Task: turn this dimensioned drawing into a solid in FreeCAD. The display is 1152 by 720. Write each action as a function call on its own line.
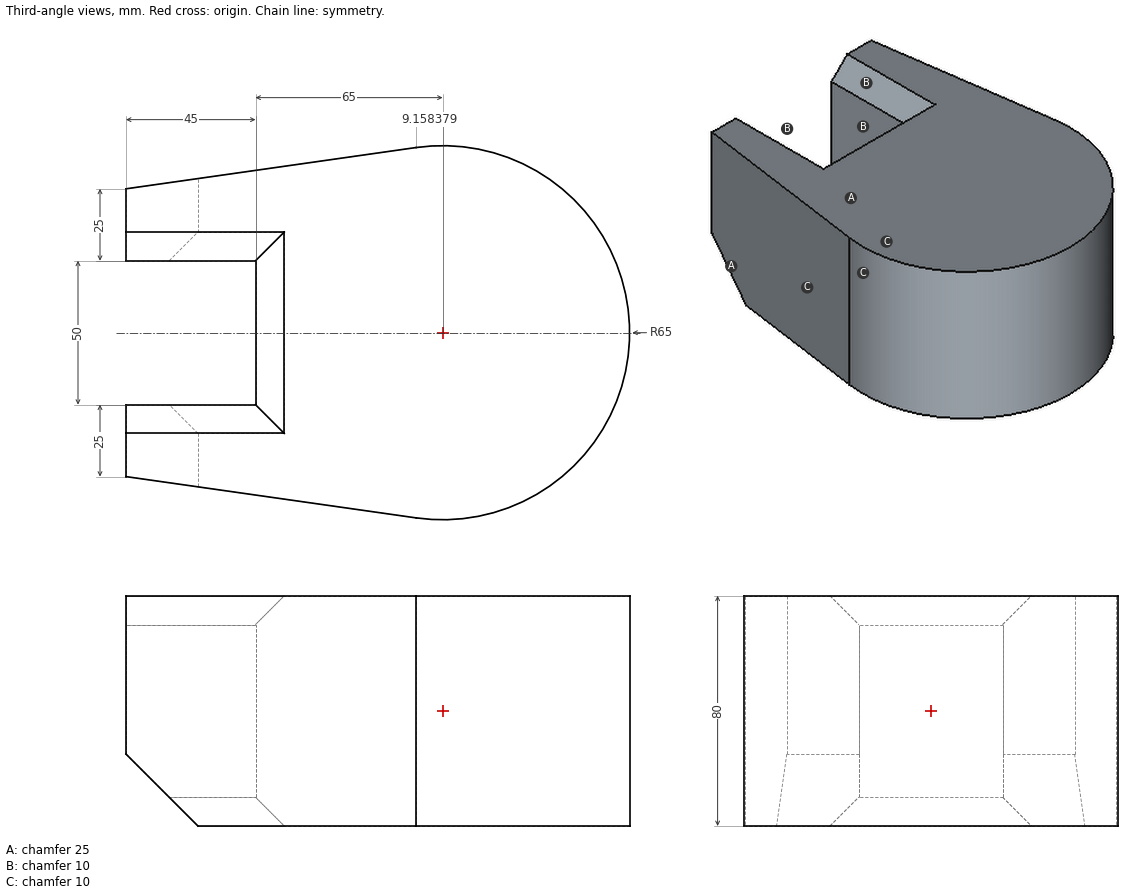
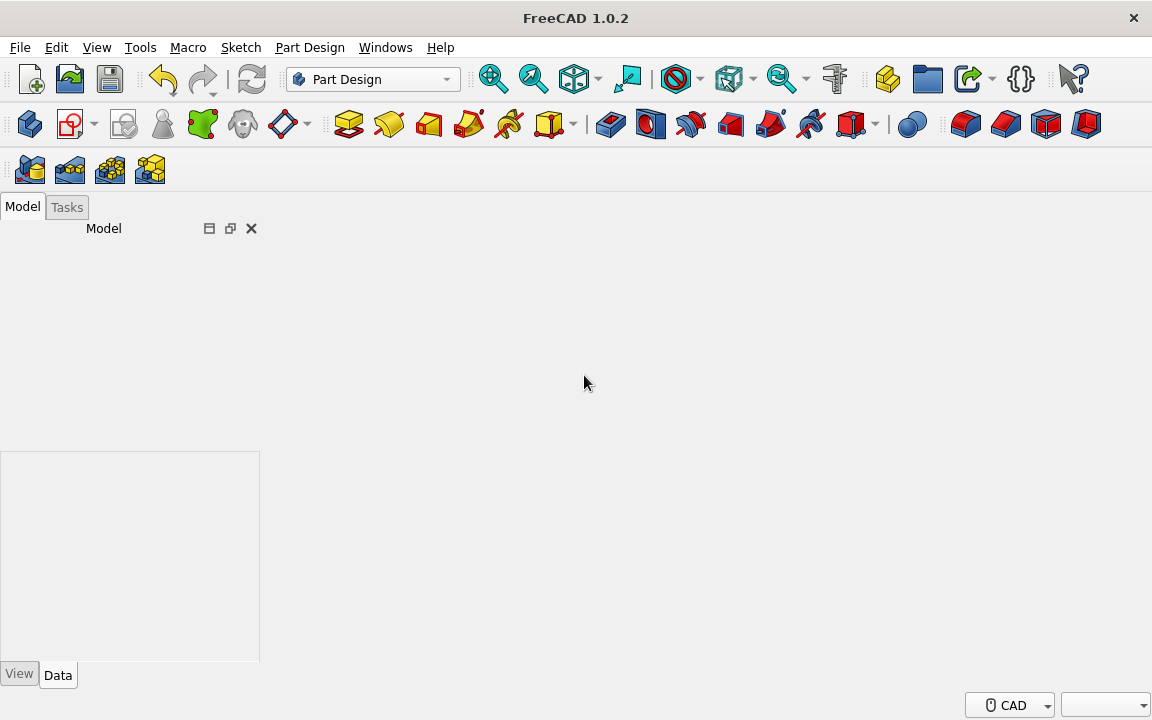
click(30, 80)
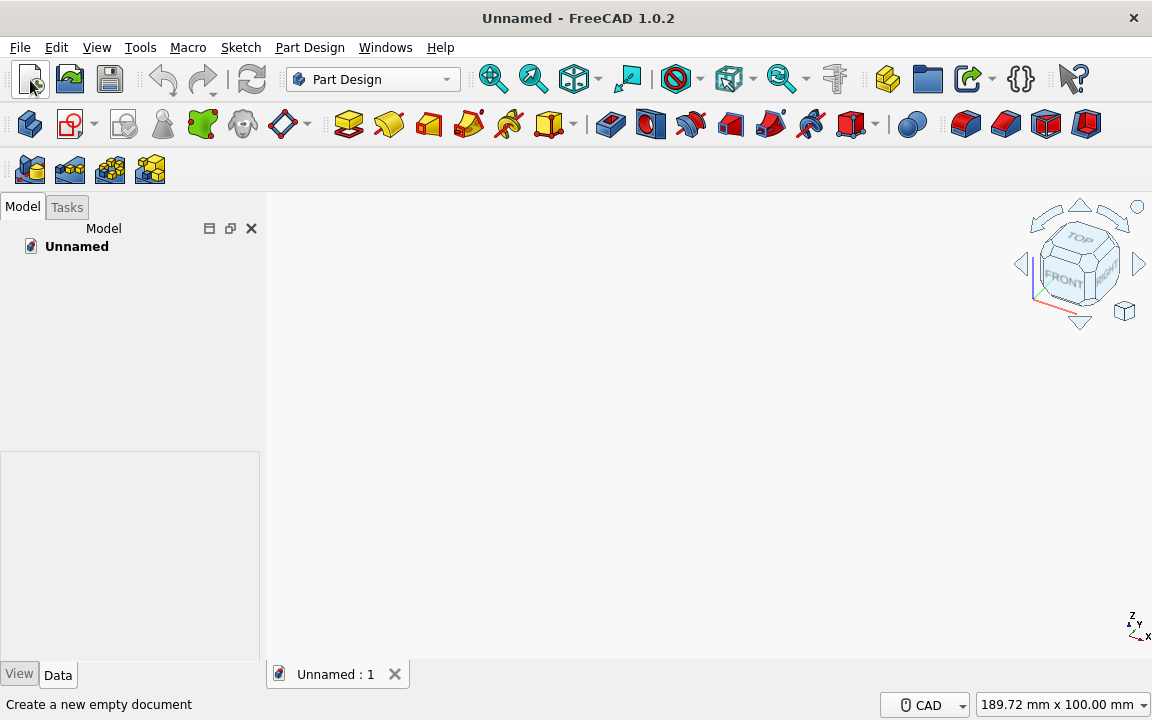
click(70, 124)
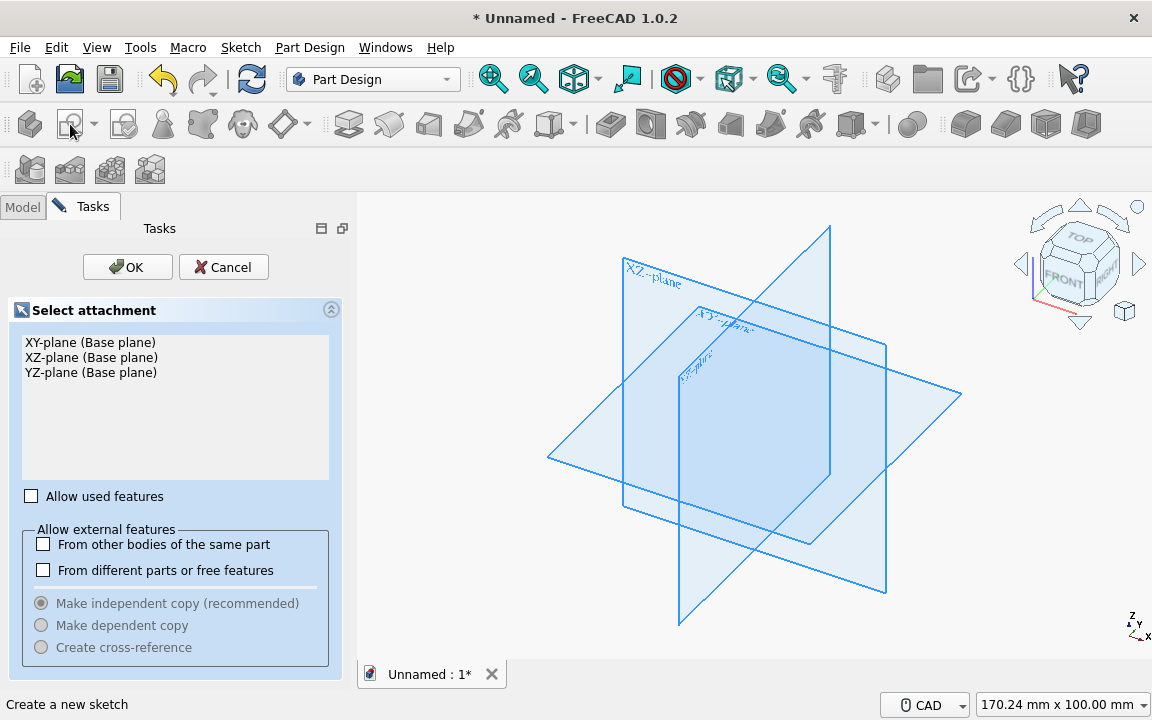
click(82, 342)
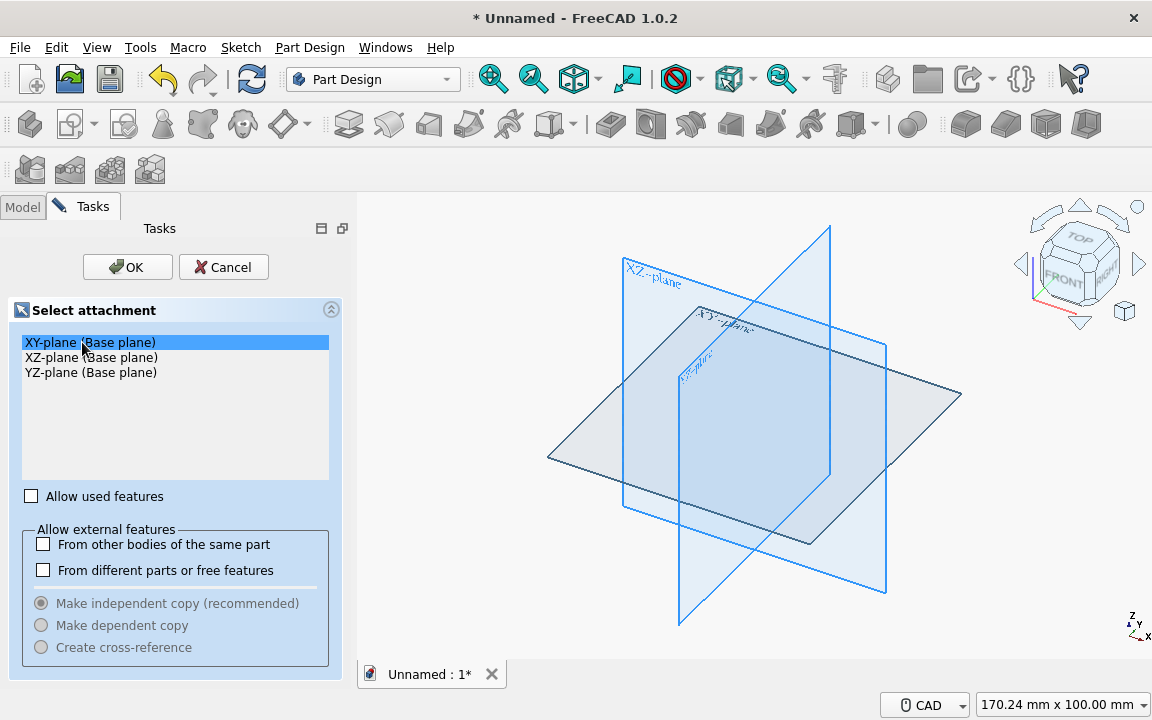
click(128, 267)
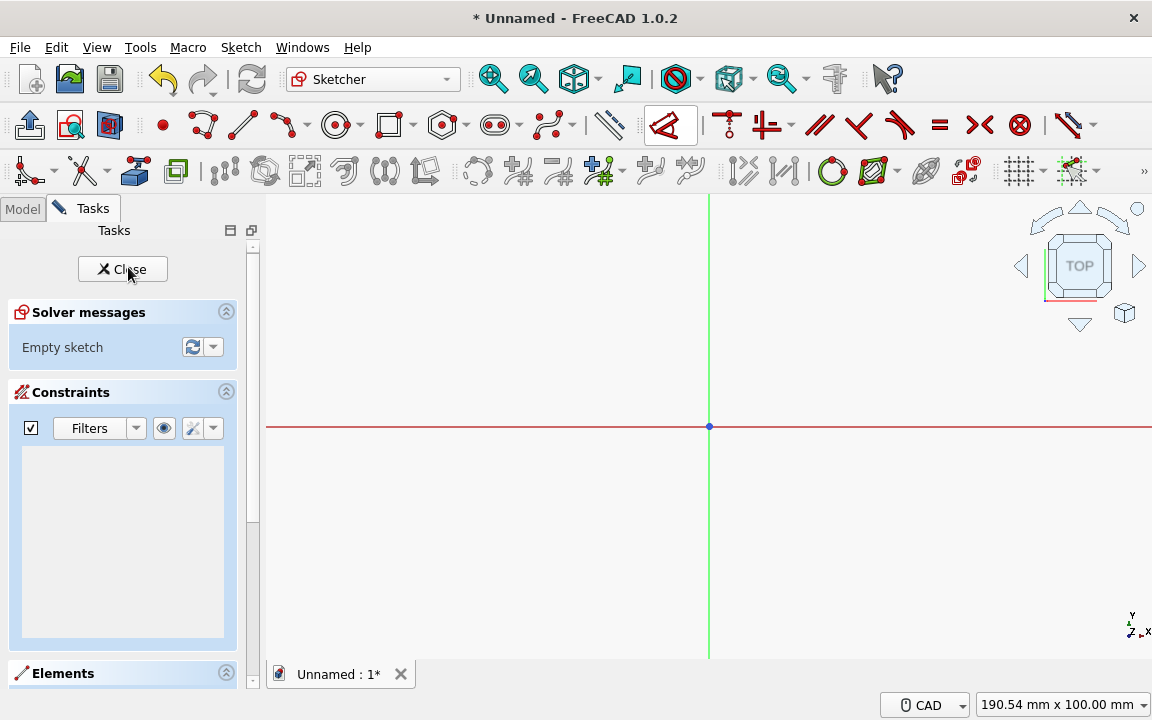
scroll(670, 426, down, 4)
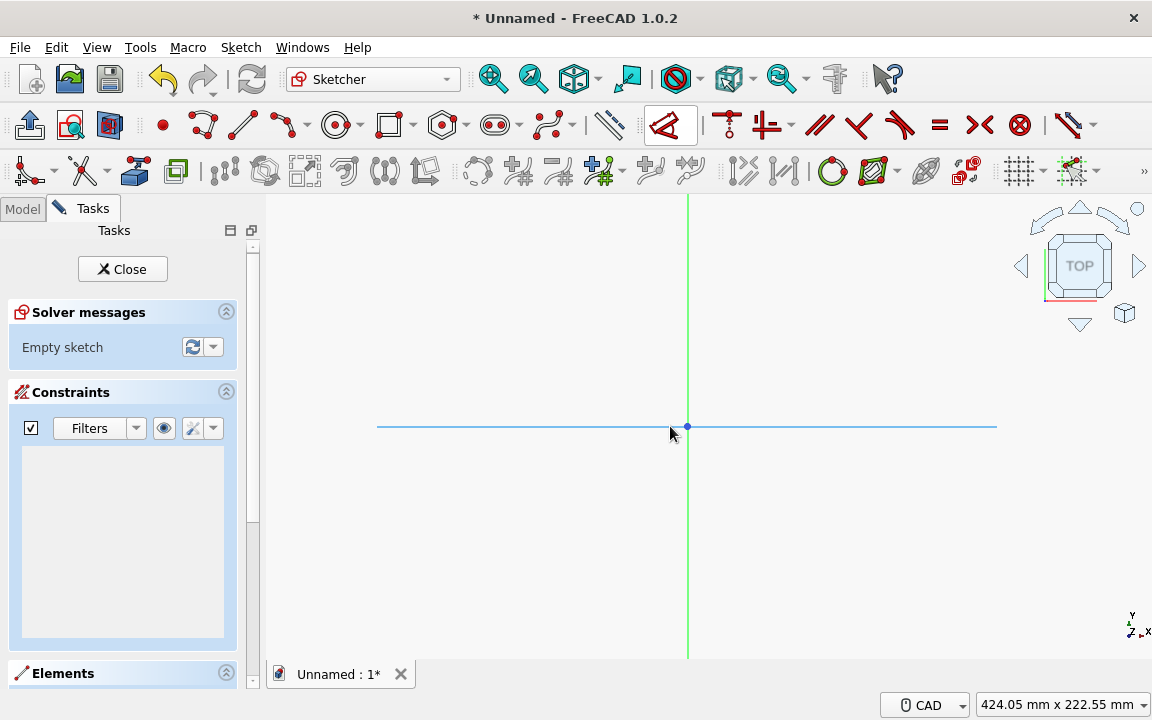
click(204, 126)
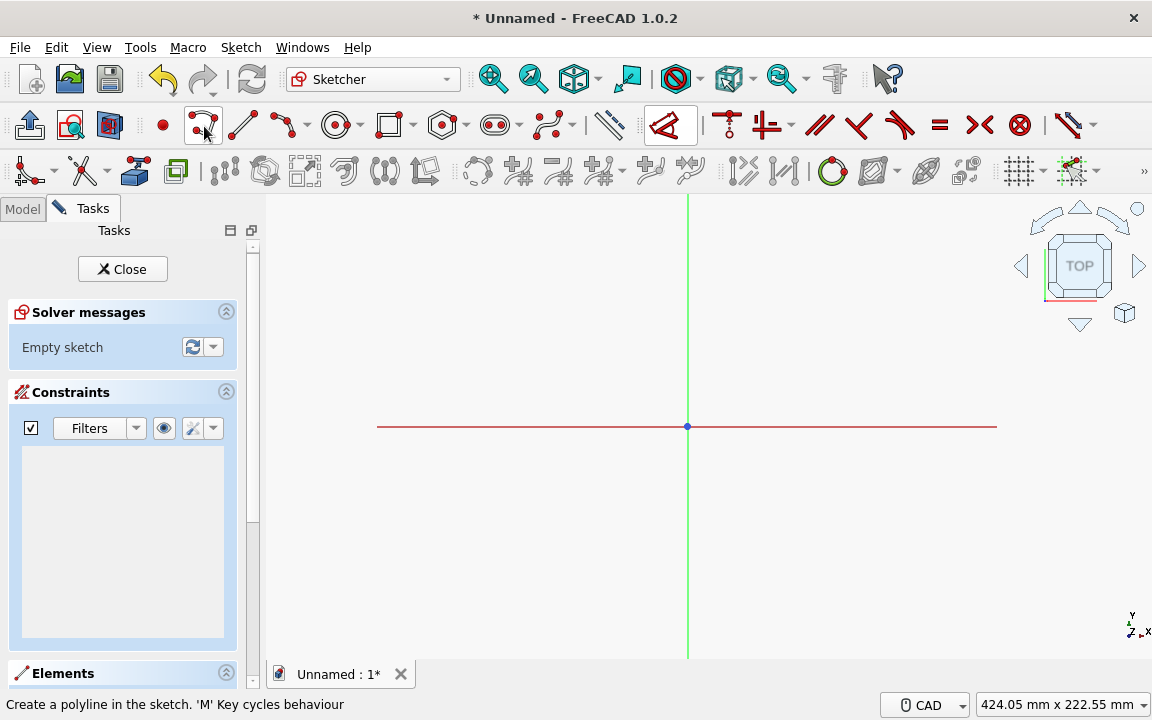
click(669, 292)
click(458, 322)
click(458, 374)
click(552, 374)
click(552, 479)
click(458, 479)
click(458, 531)
click(669, 561)
right_click(669, 561)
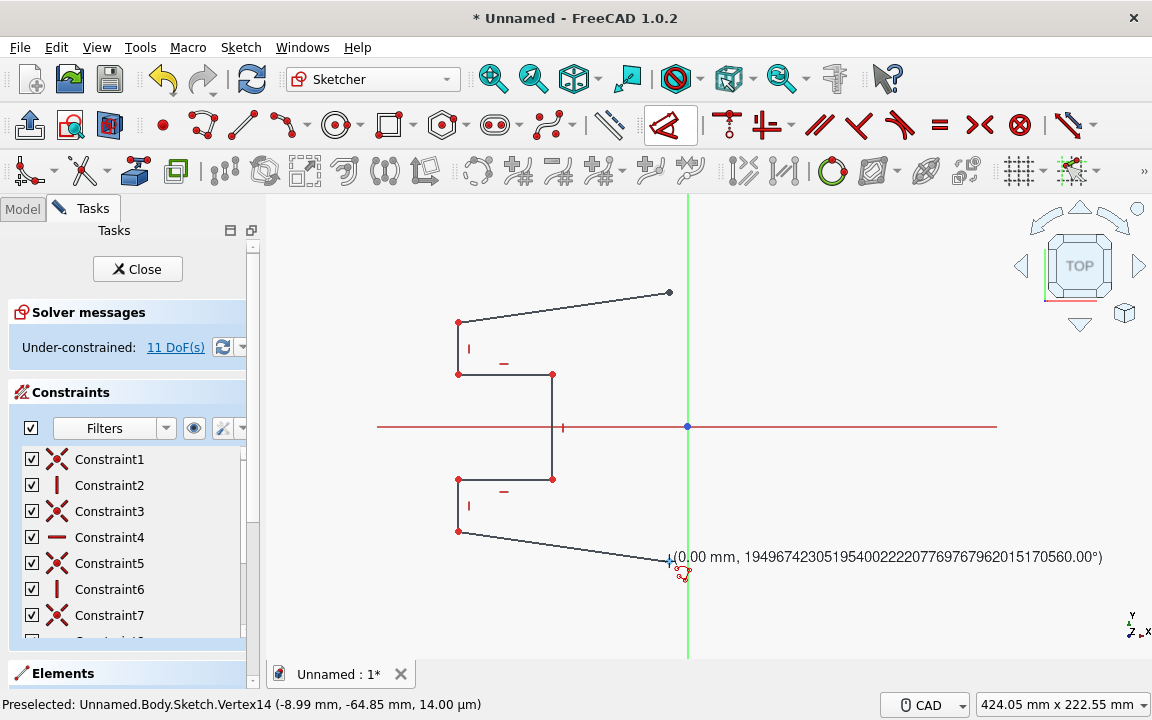
click(284, 126)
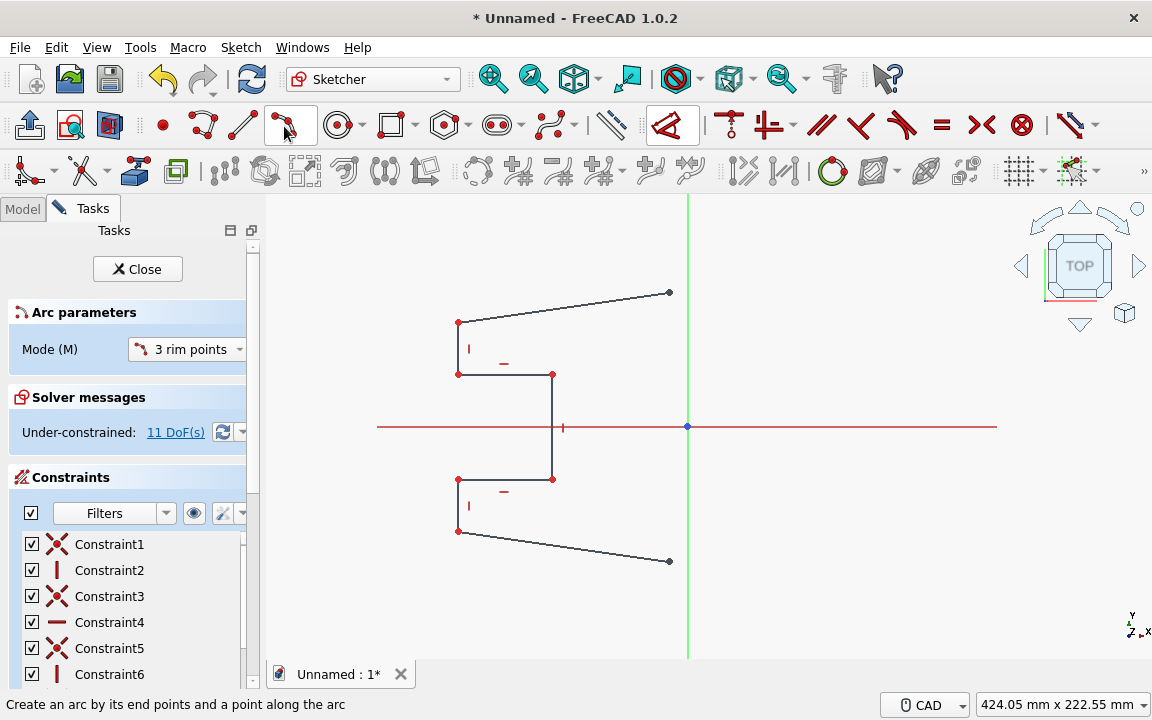
click(669, 562)
click(669, 293)
click(816, 472)
key(Escape)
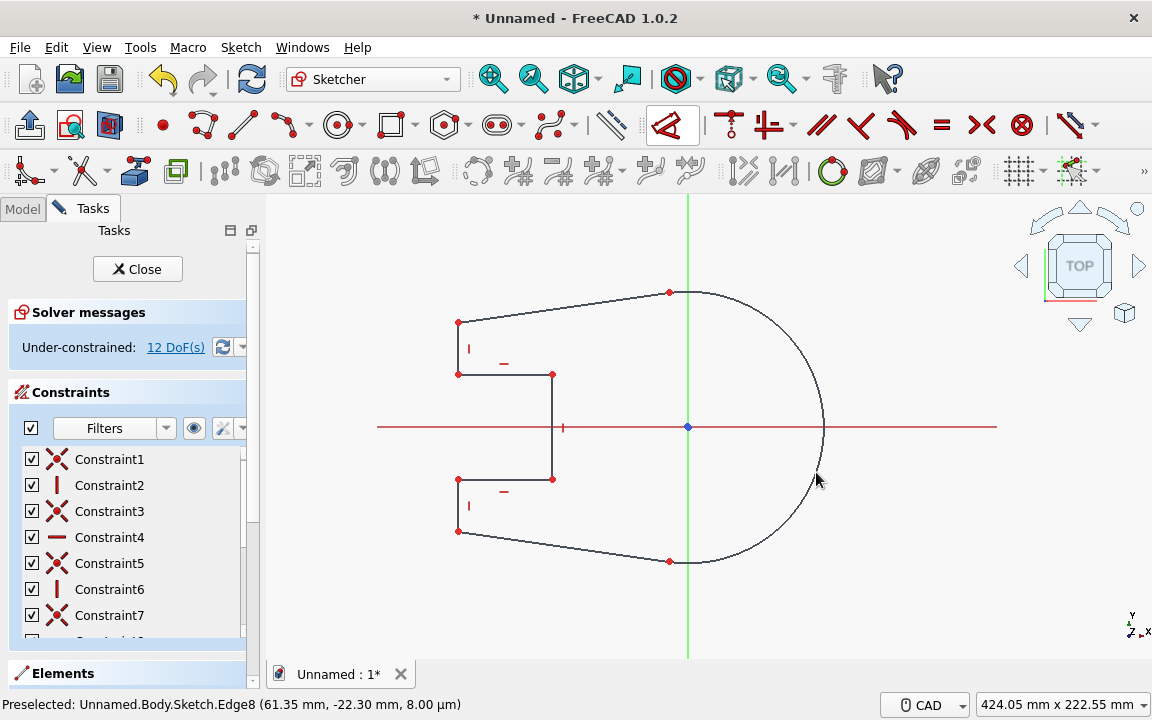
drag(678, 416, 698, 438)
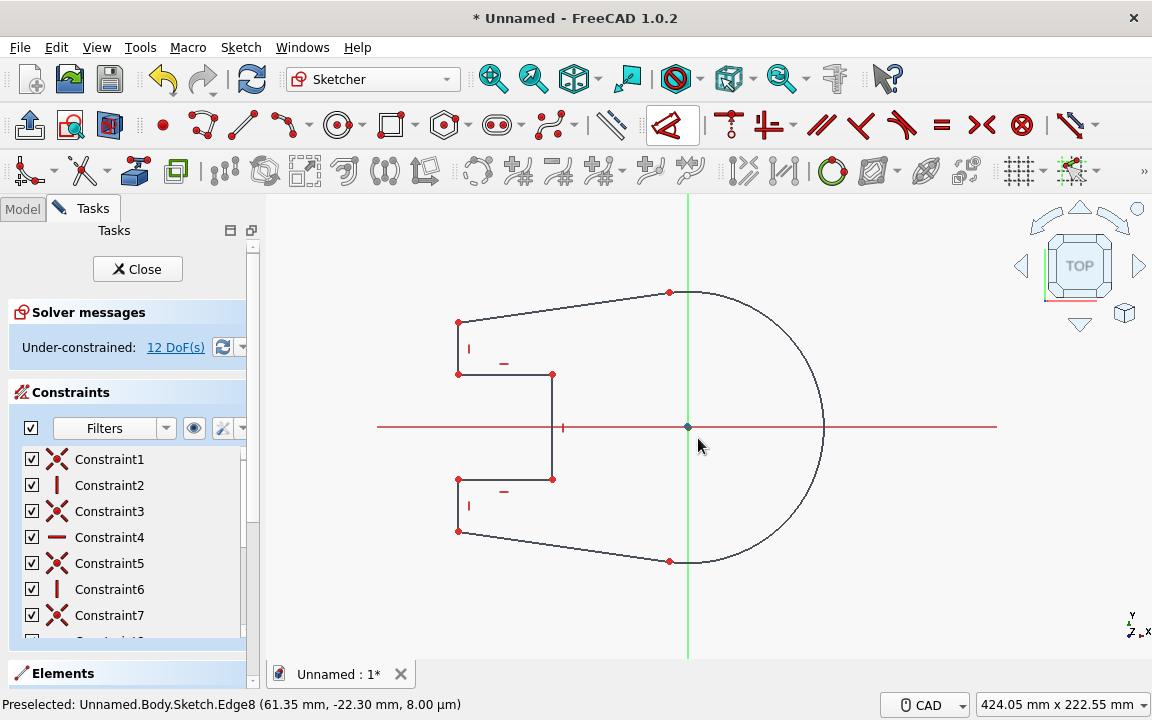
key(c)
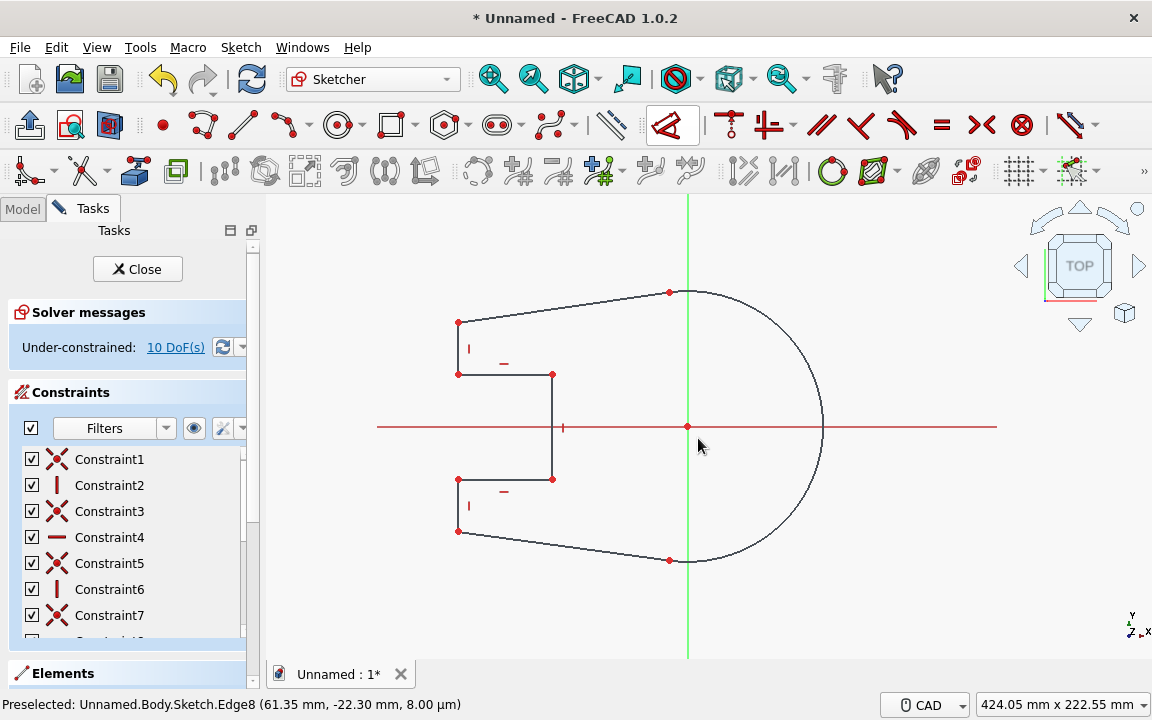
click(458, 375)